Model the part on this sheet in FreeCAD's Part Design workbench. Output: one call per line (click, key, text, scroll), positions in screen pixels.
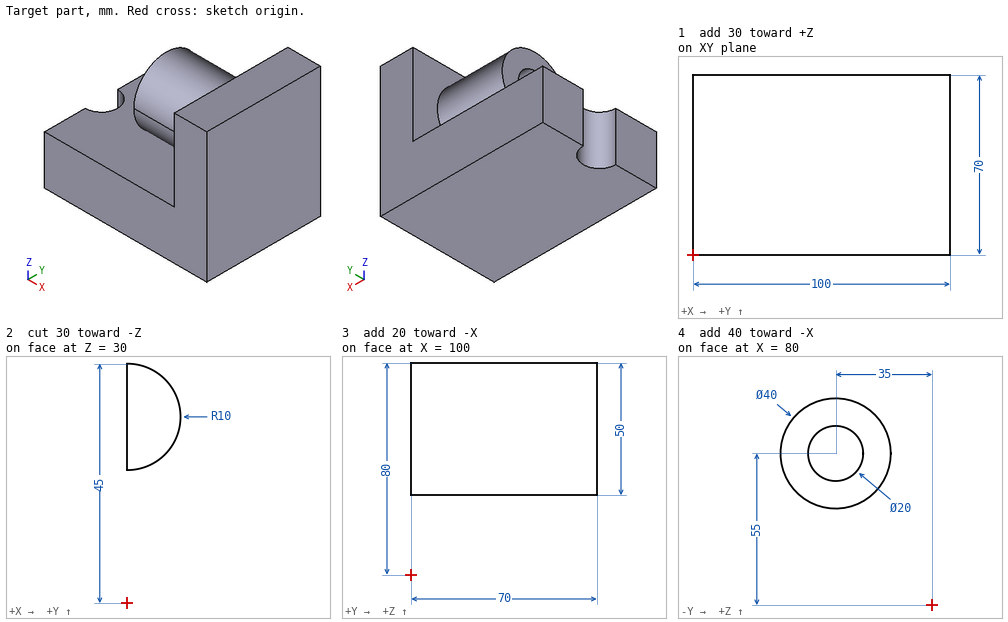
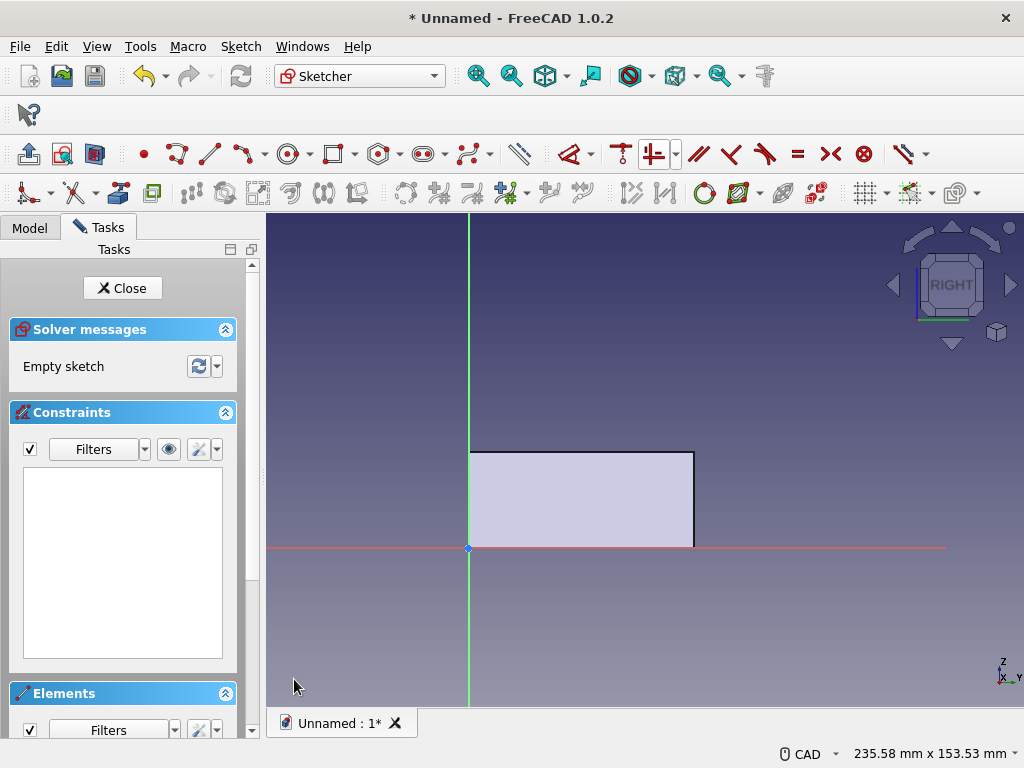
click(332, 154)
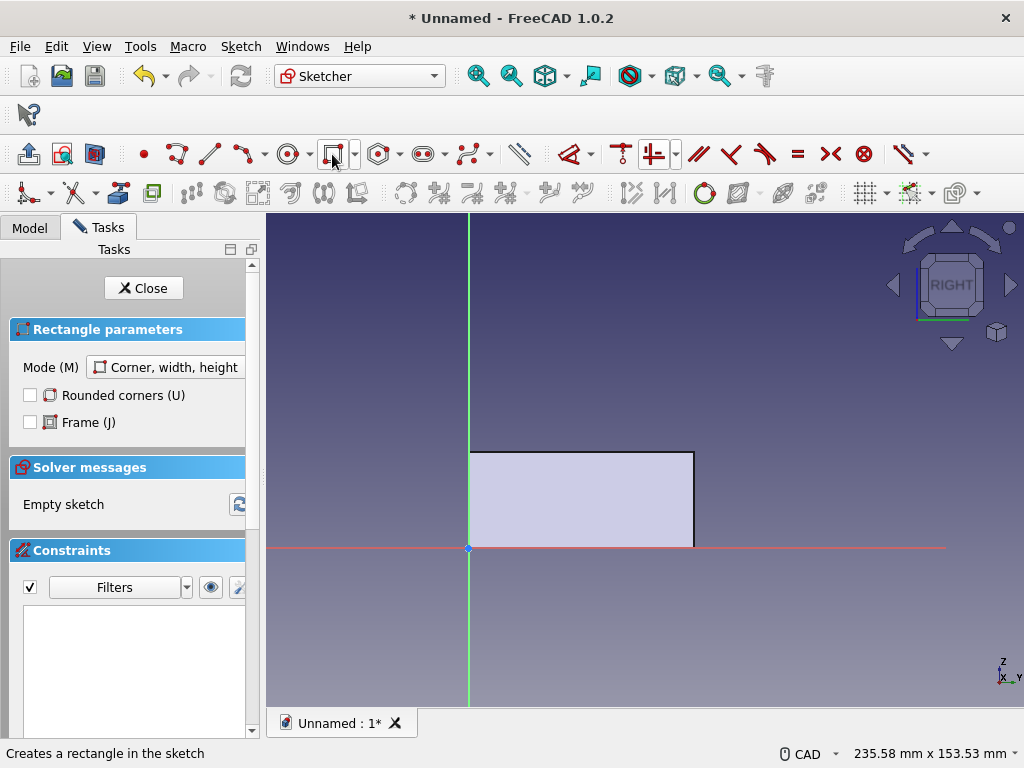
click(469, 291)
move(694, 452)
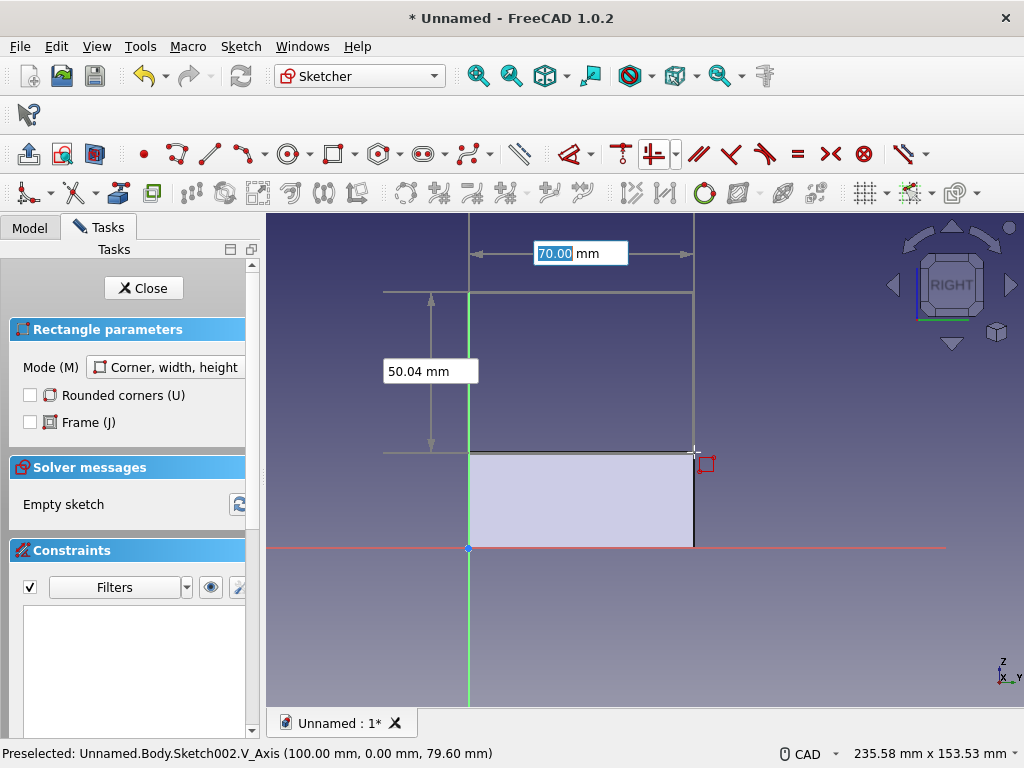
text(70)
key(Tab)
text(50)
key(Return)
key(Escape)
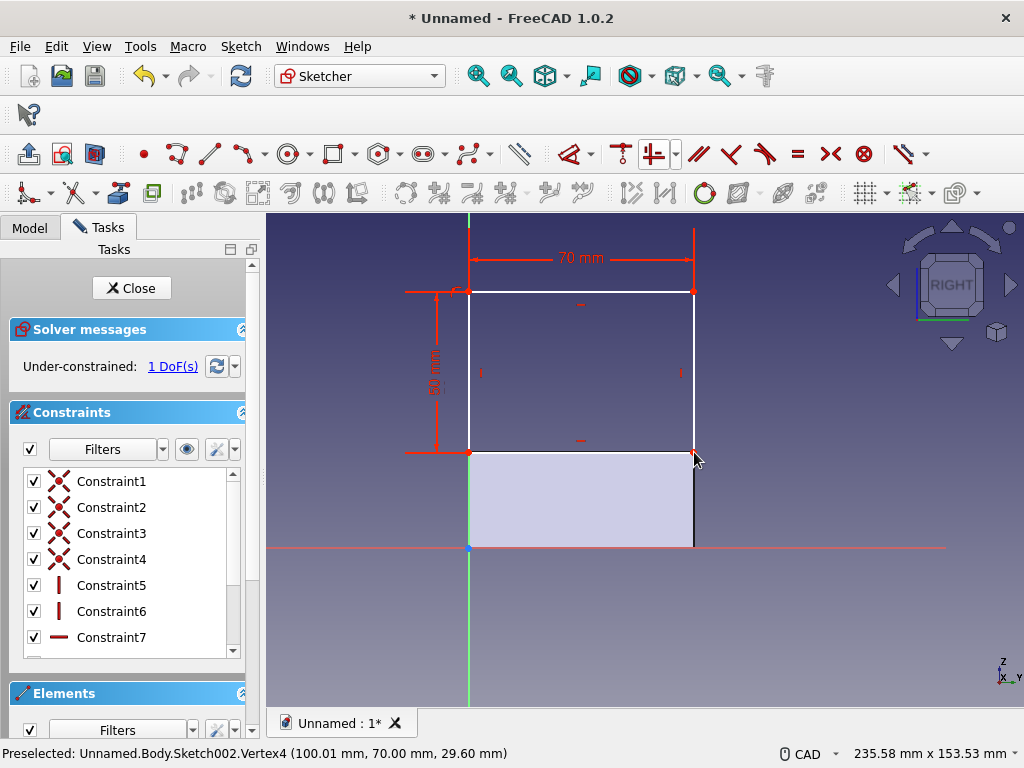
key(d)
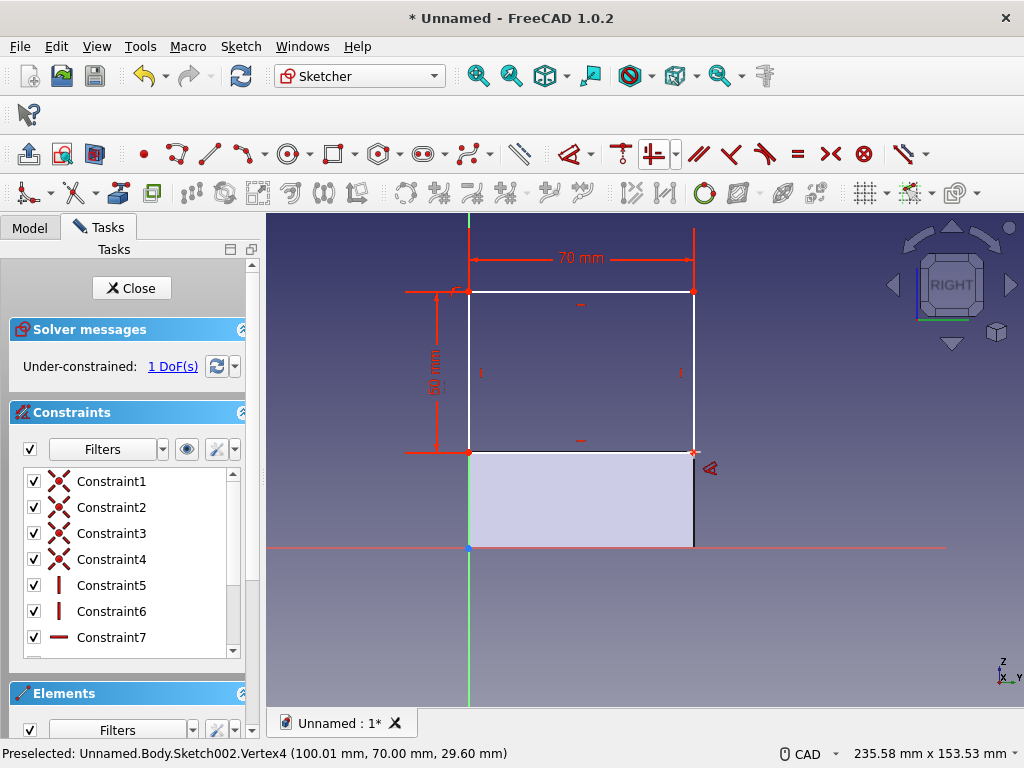
click(469, 292)
click(435, 420)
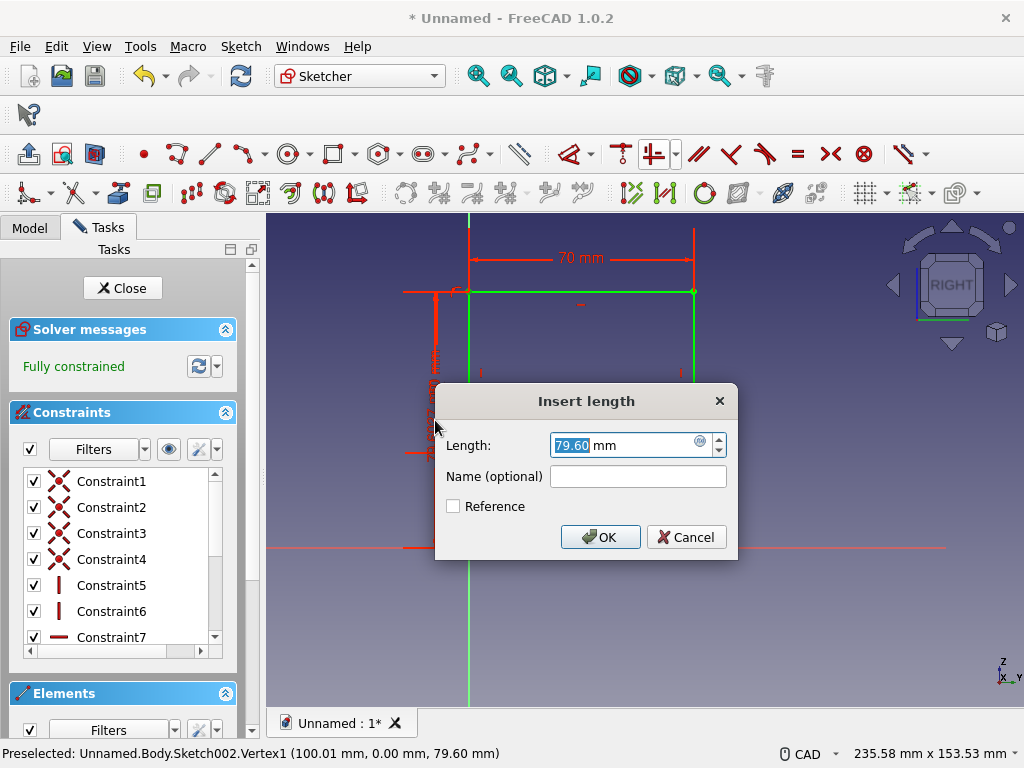
text(80)
key(Return)
key(Escape)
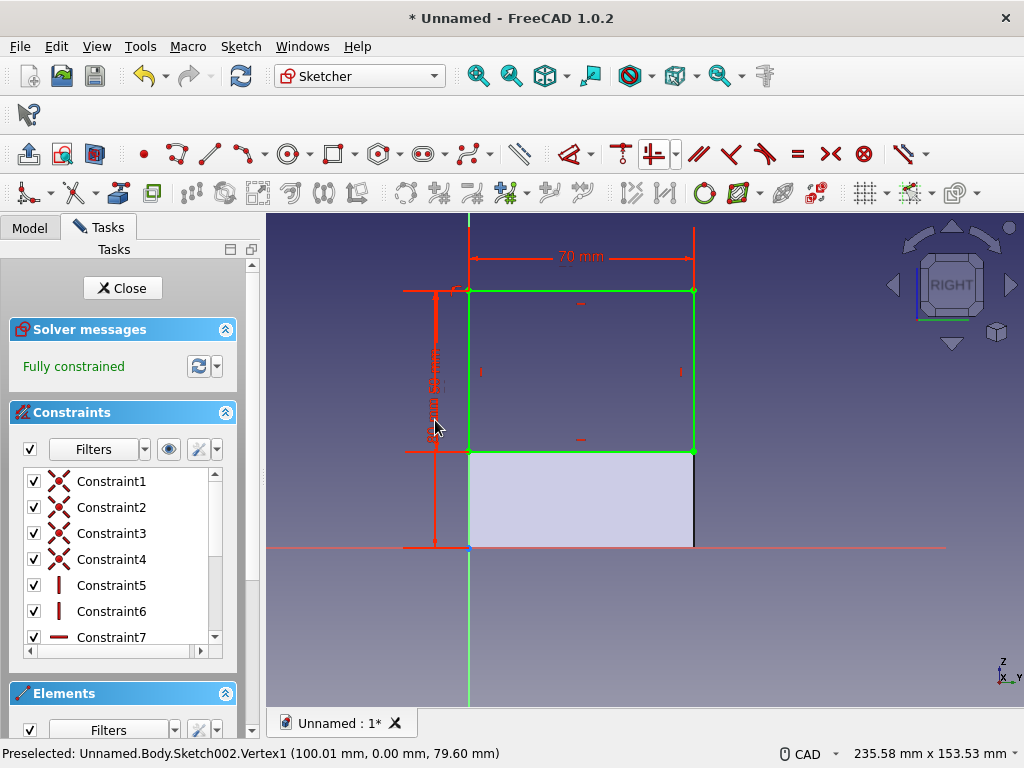
click(123, 288)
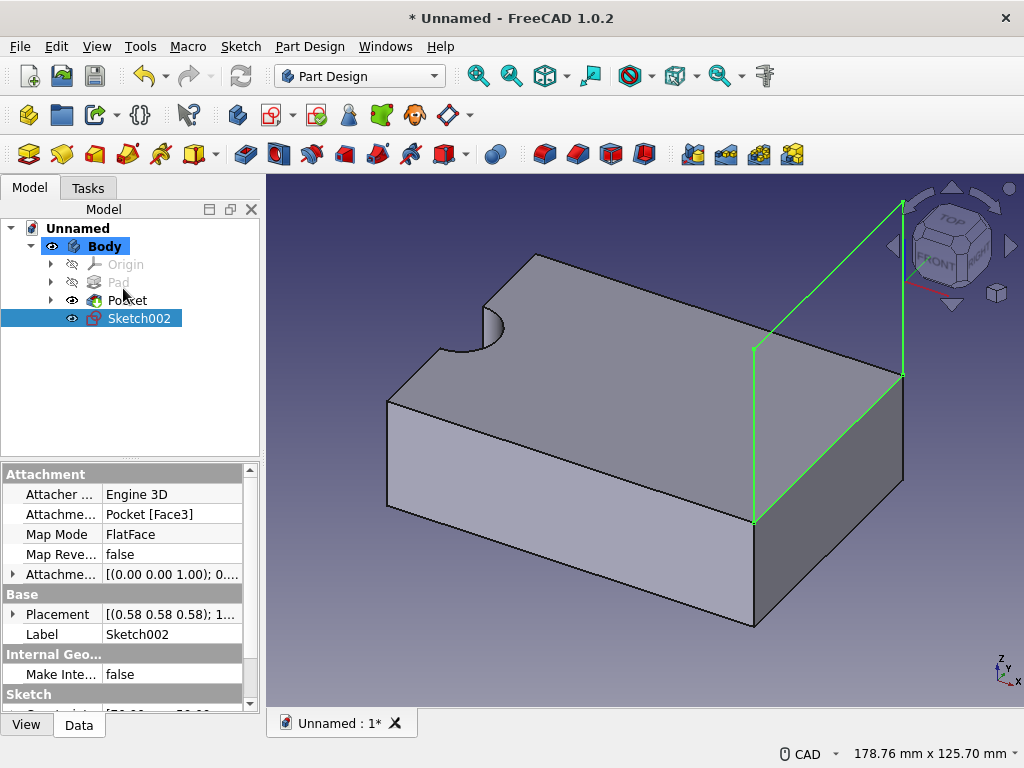
click(29, 154)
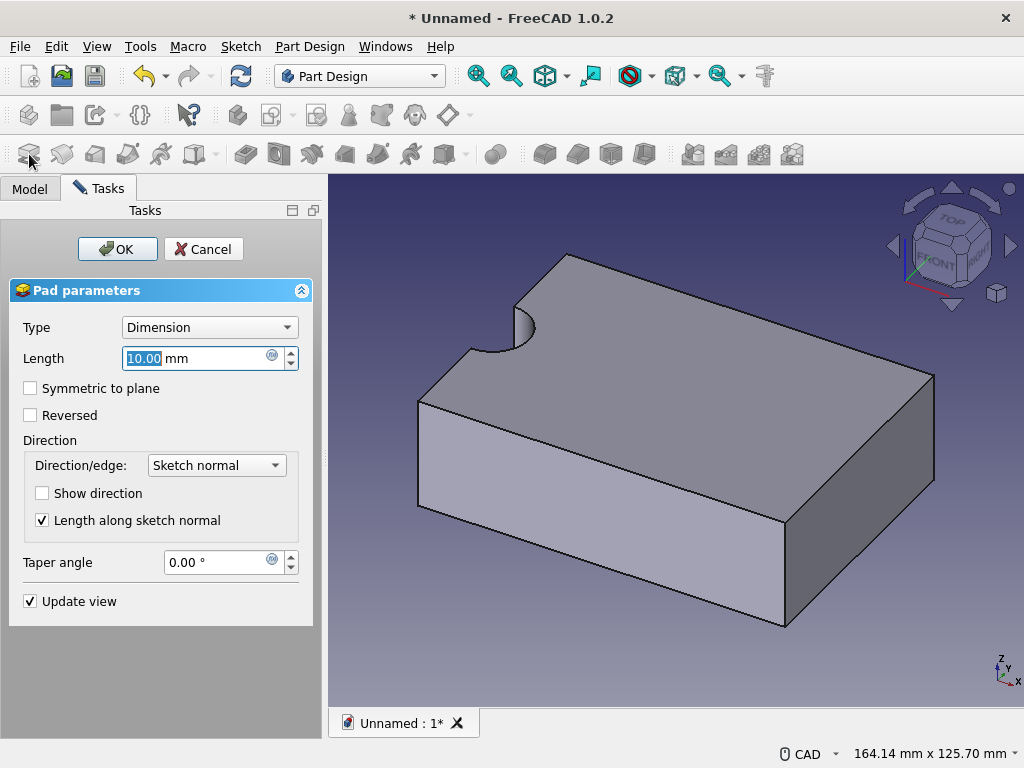
text(20)
key(Tab)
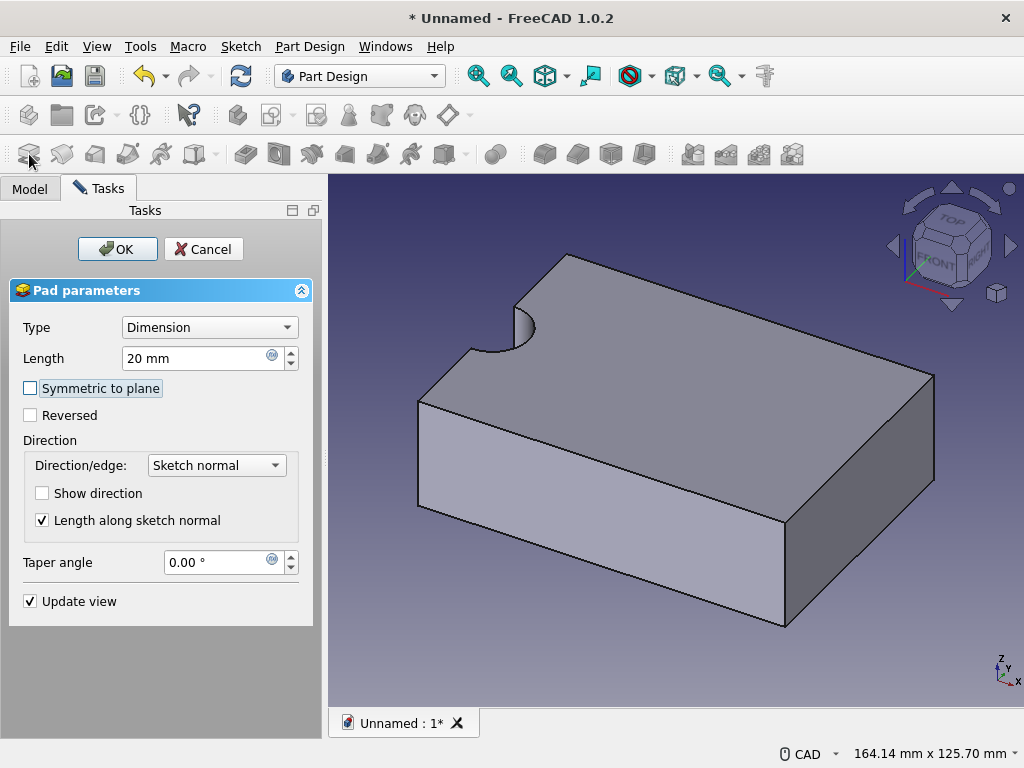
click(31, 415)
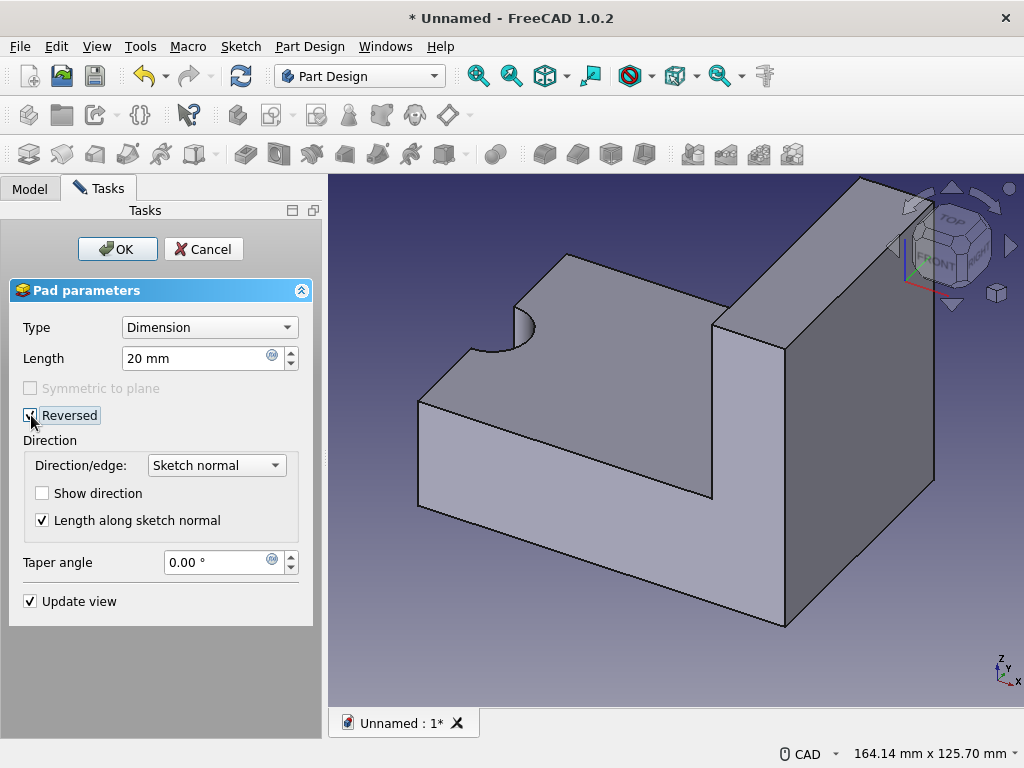
click(118, 249)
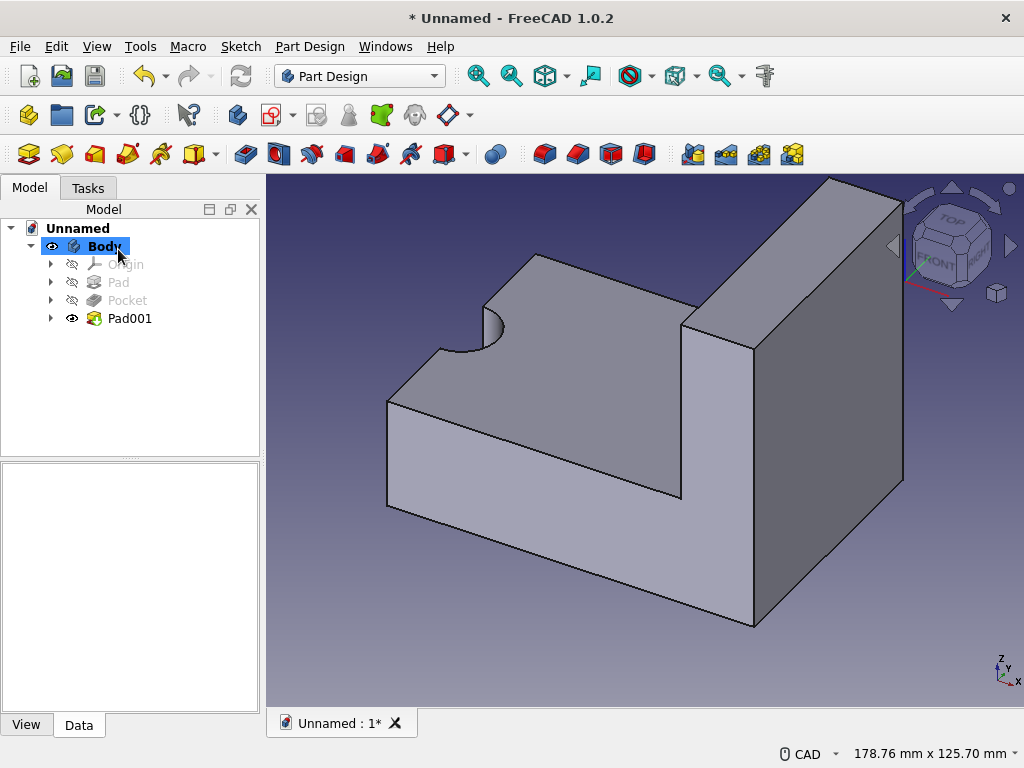
click(479, 76)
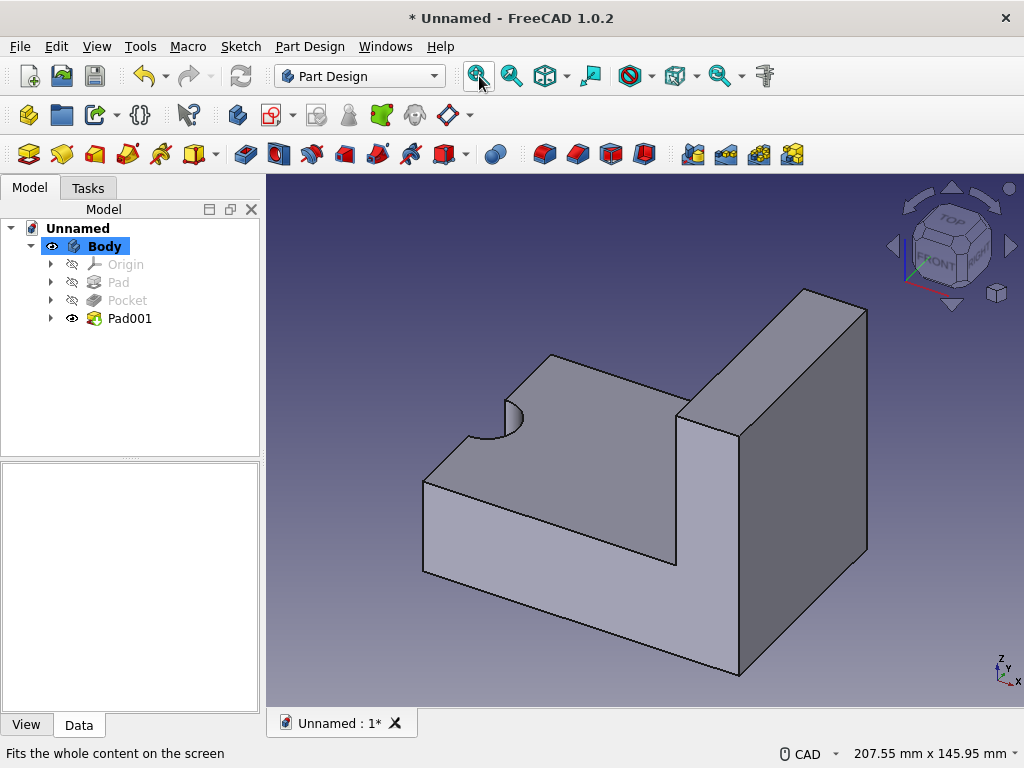
key(6)